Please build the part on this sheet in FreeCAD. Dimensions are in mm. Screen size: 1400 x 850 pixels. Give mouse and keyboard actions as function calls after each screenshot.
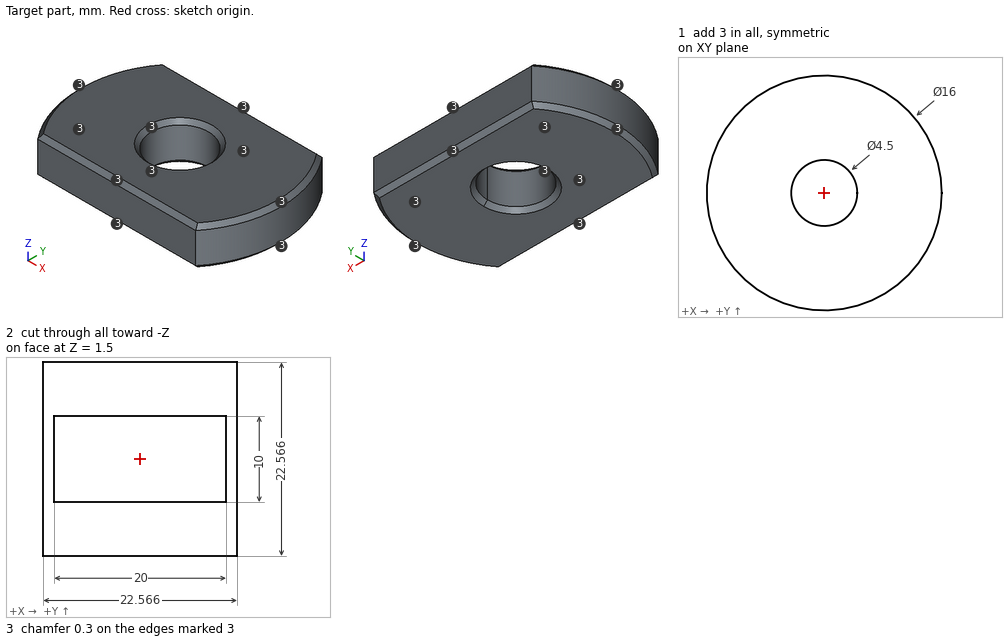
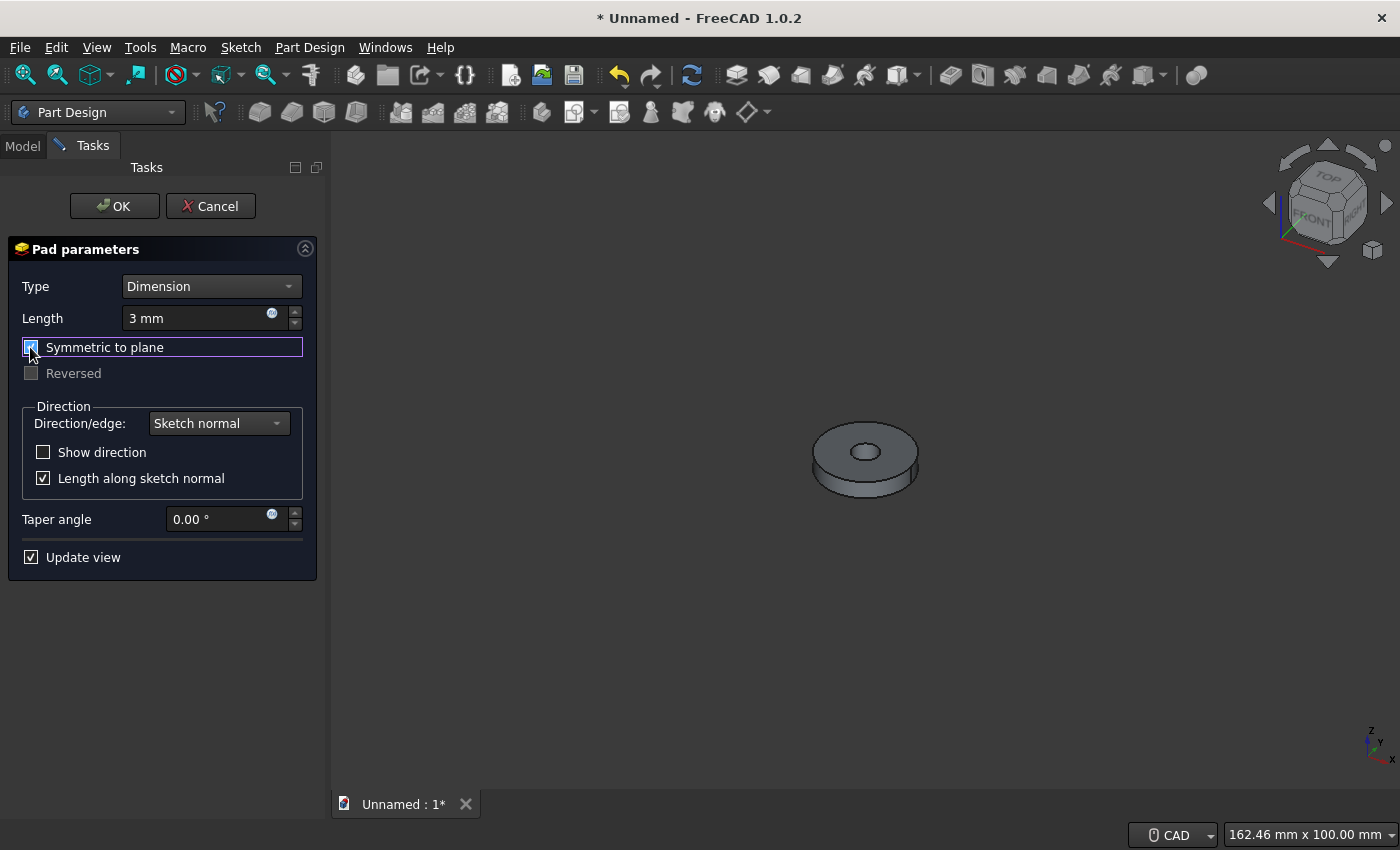
click(115, 206)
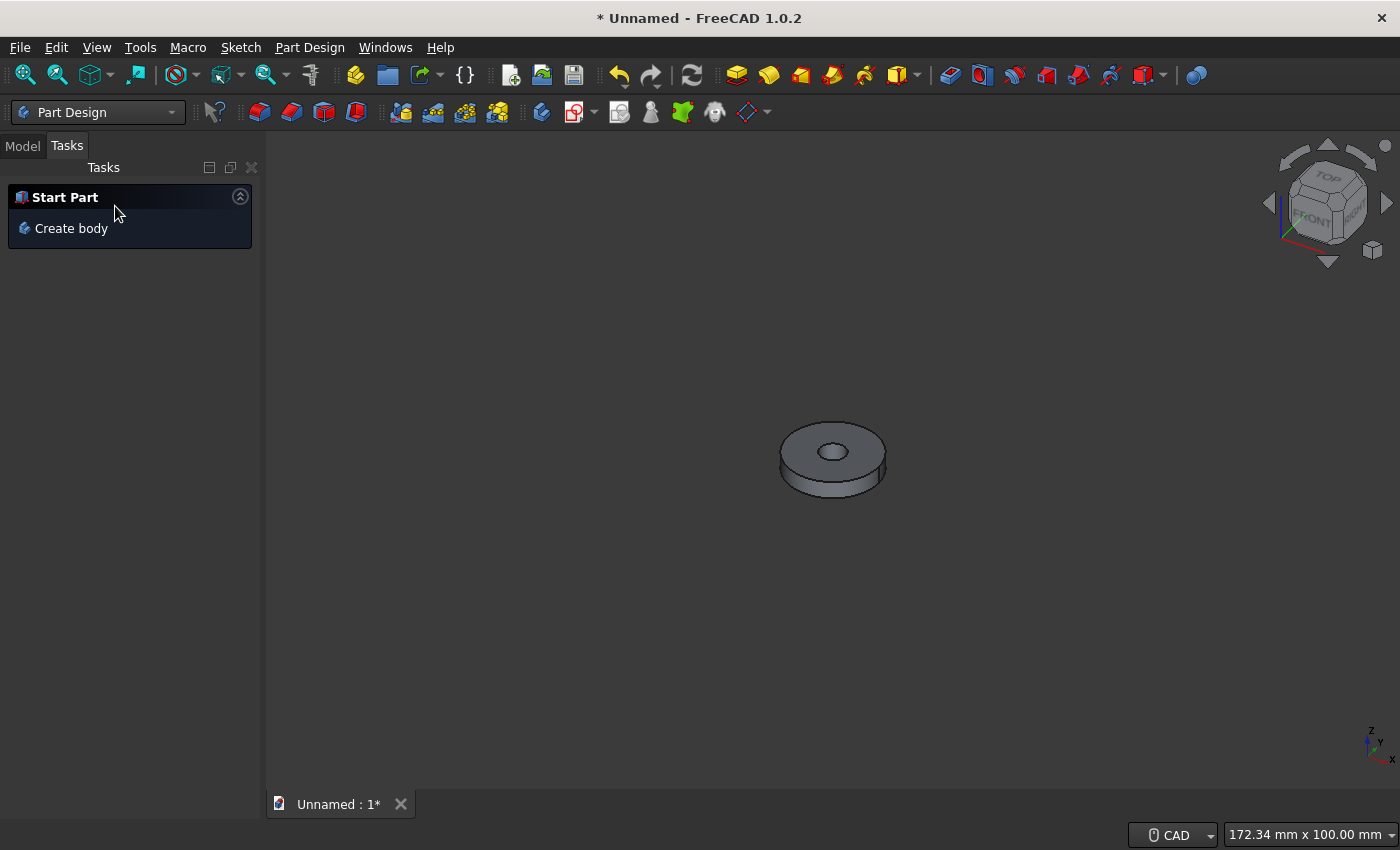
click(26, 76)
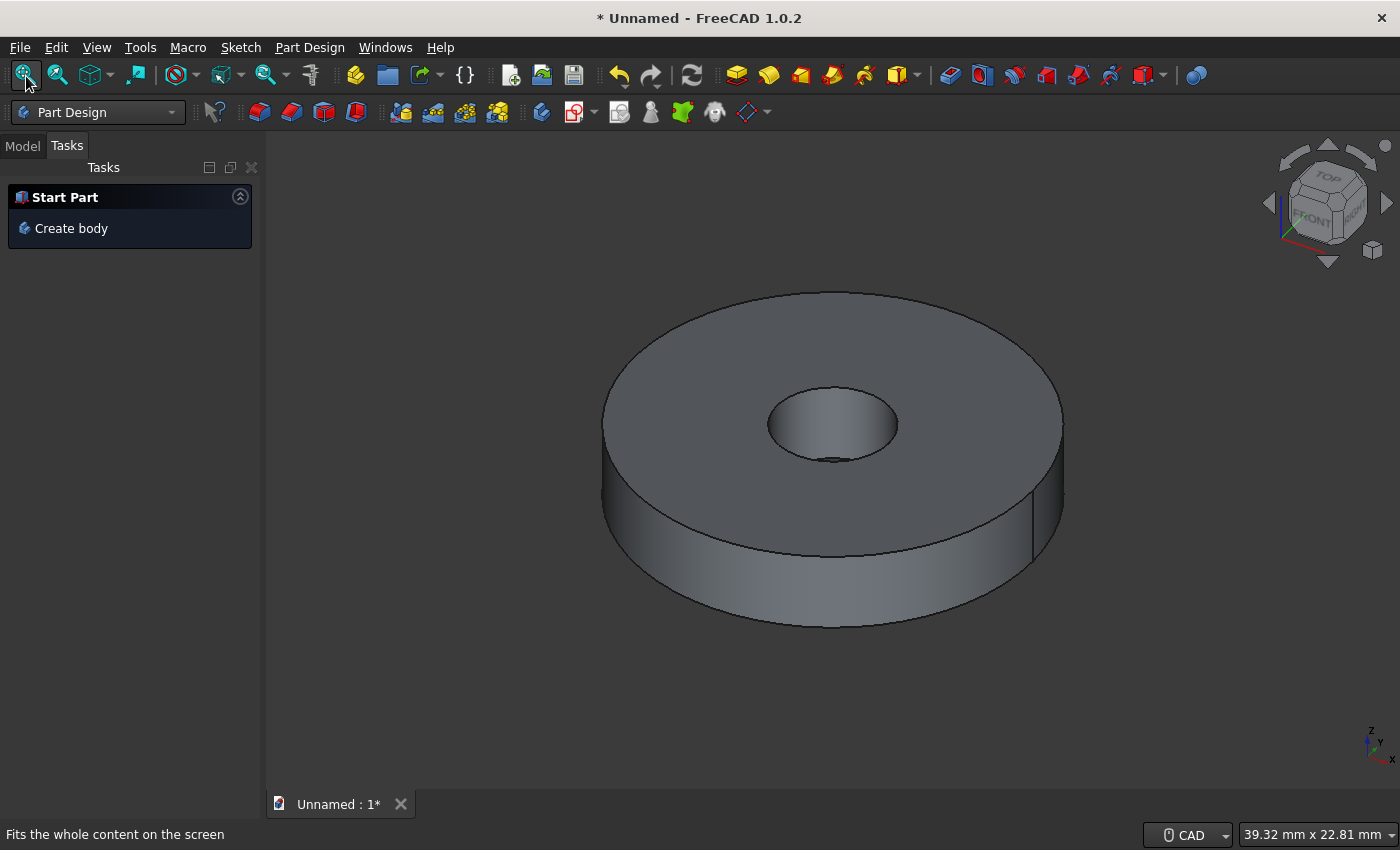
click(956, 377)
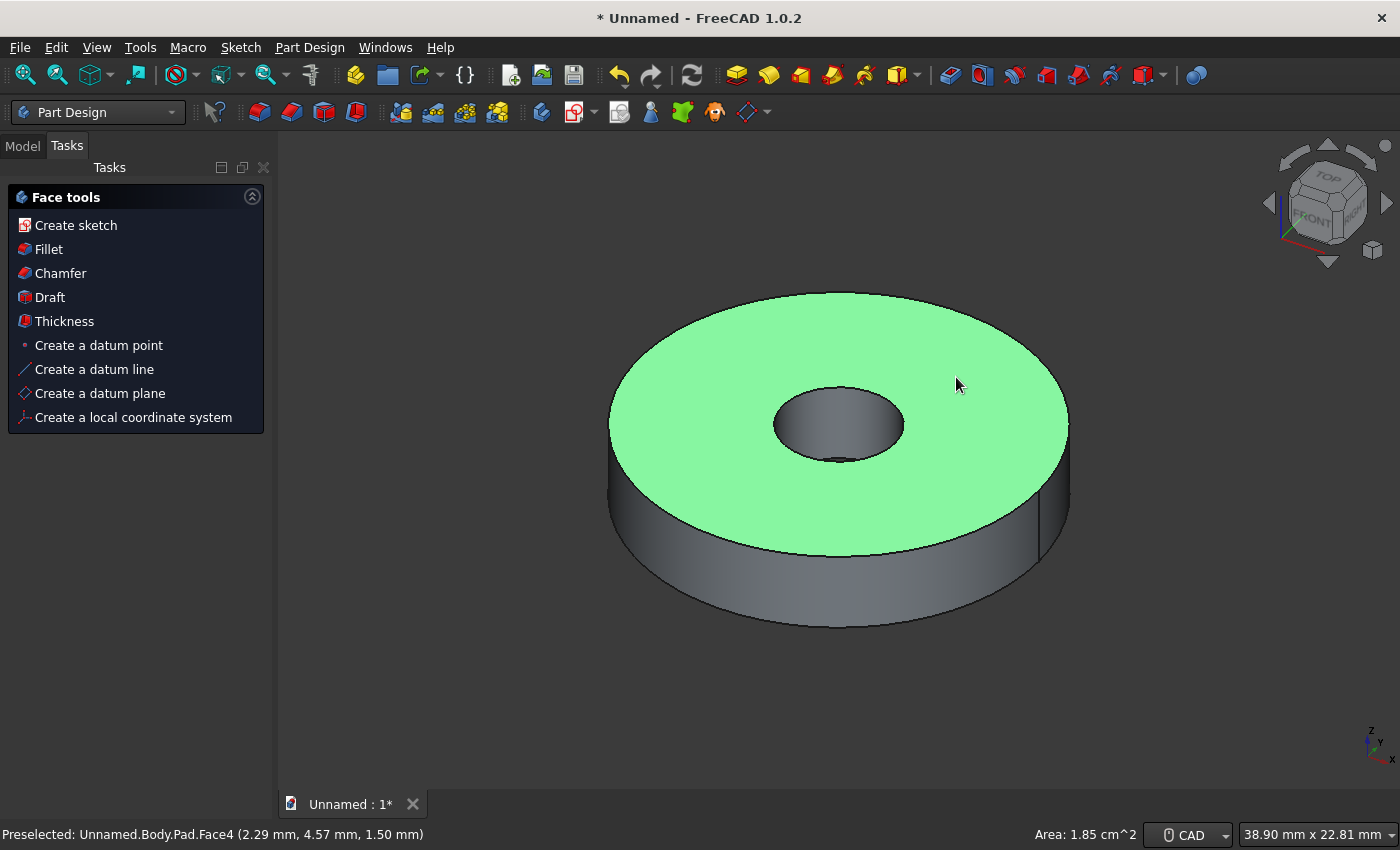
click(574, 112)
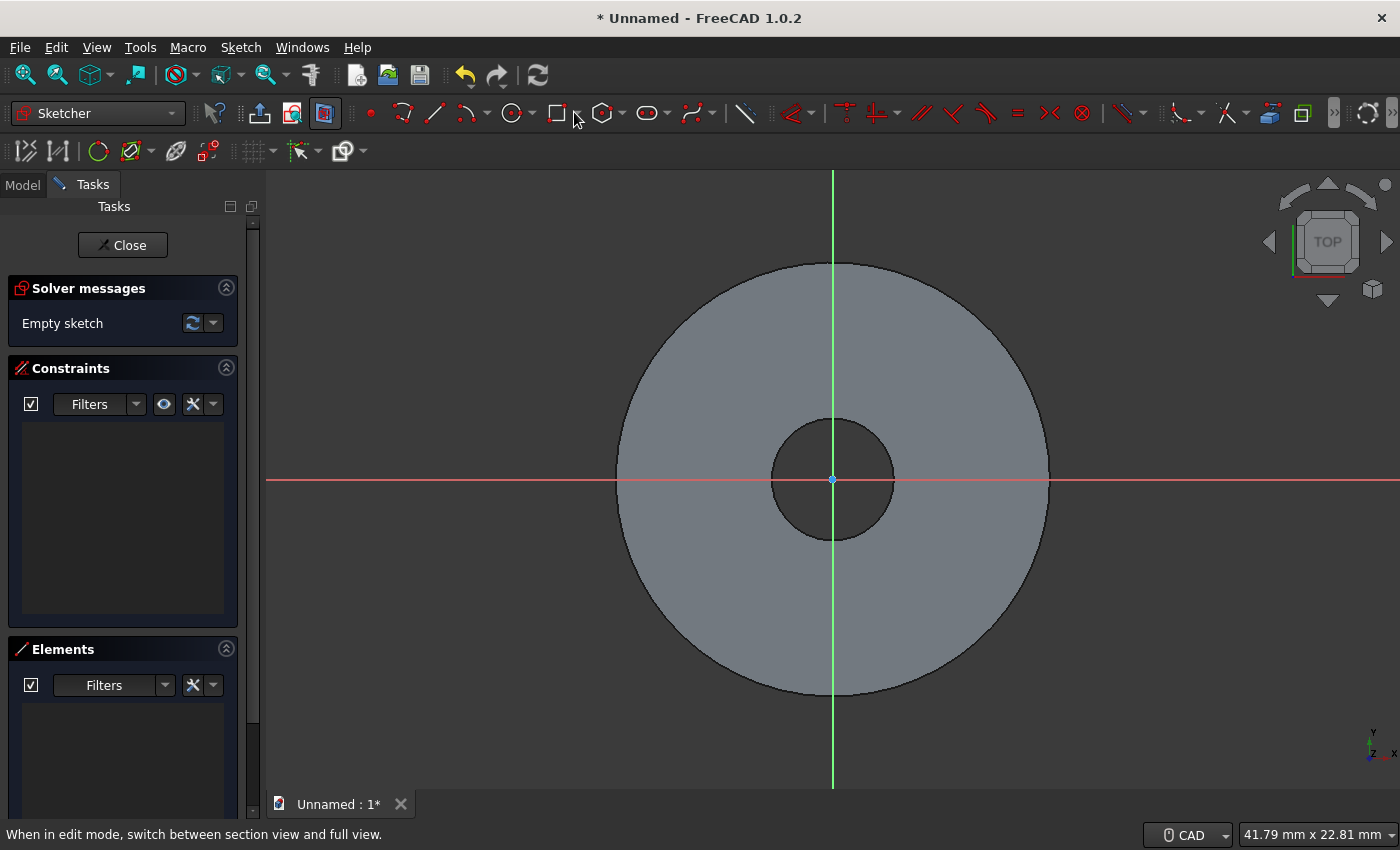
scroll(626, 480, down, 2)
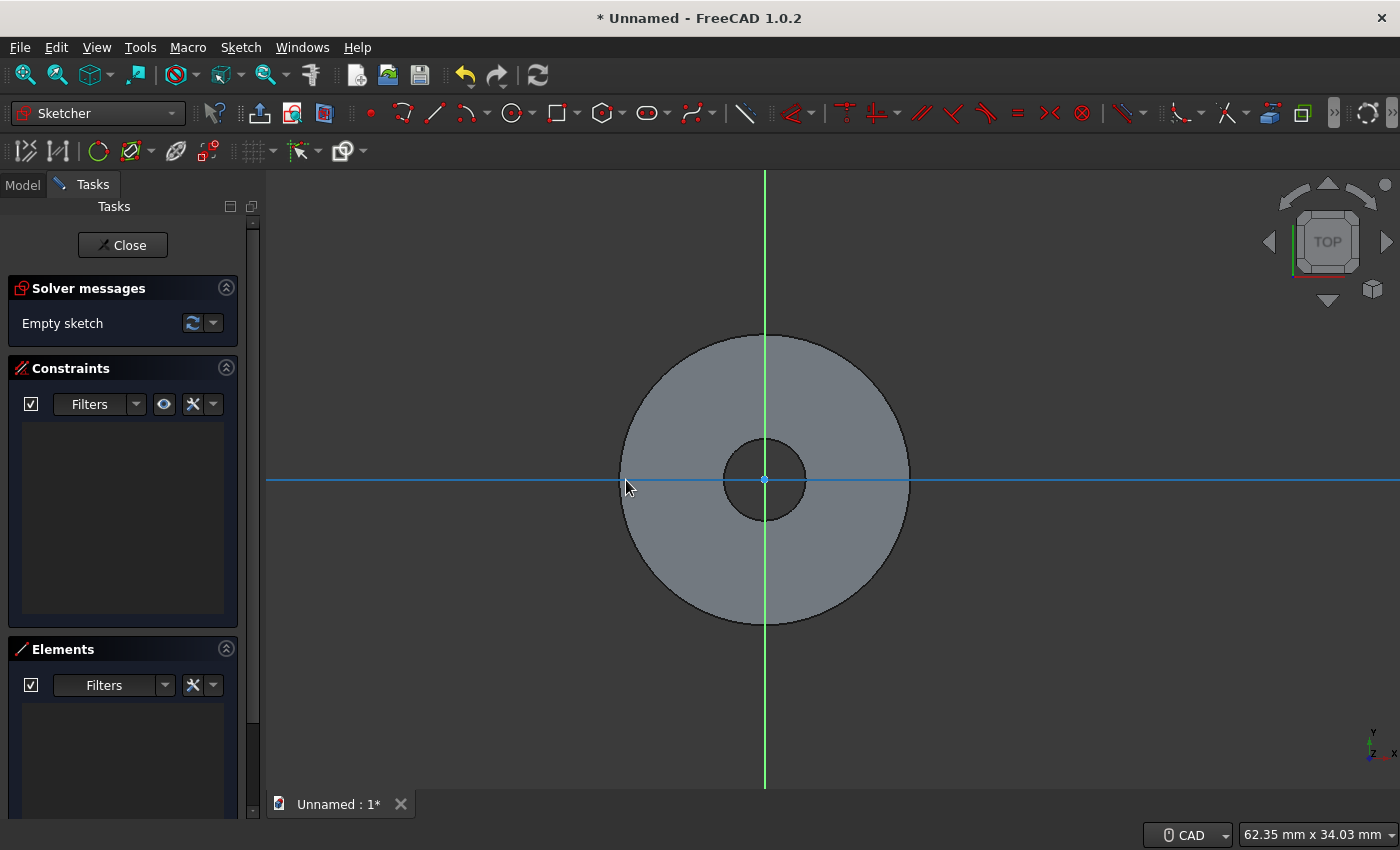
click(580, 114)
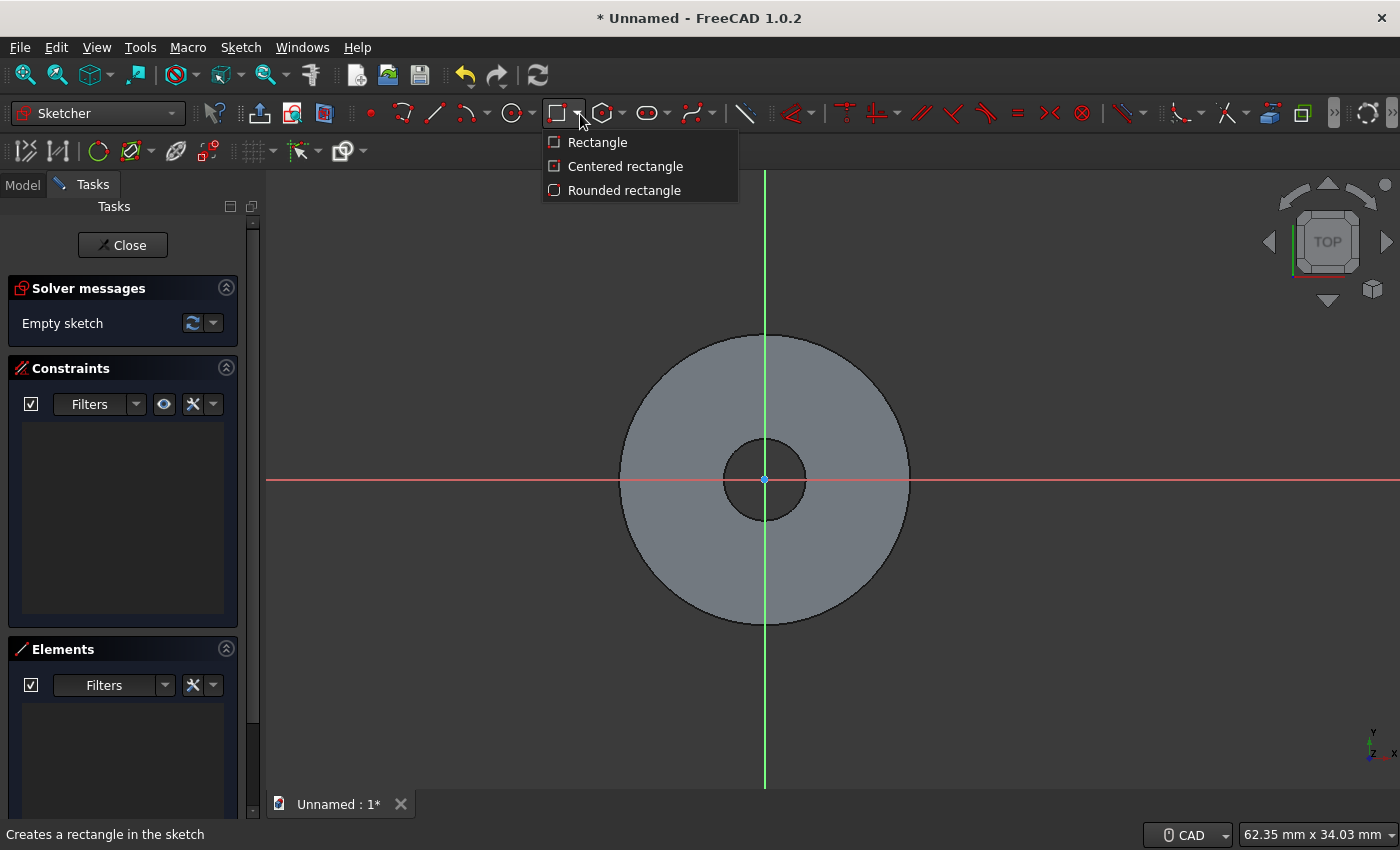
click(640, 166)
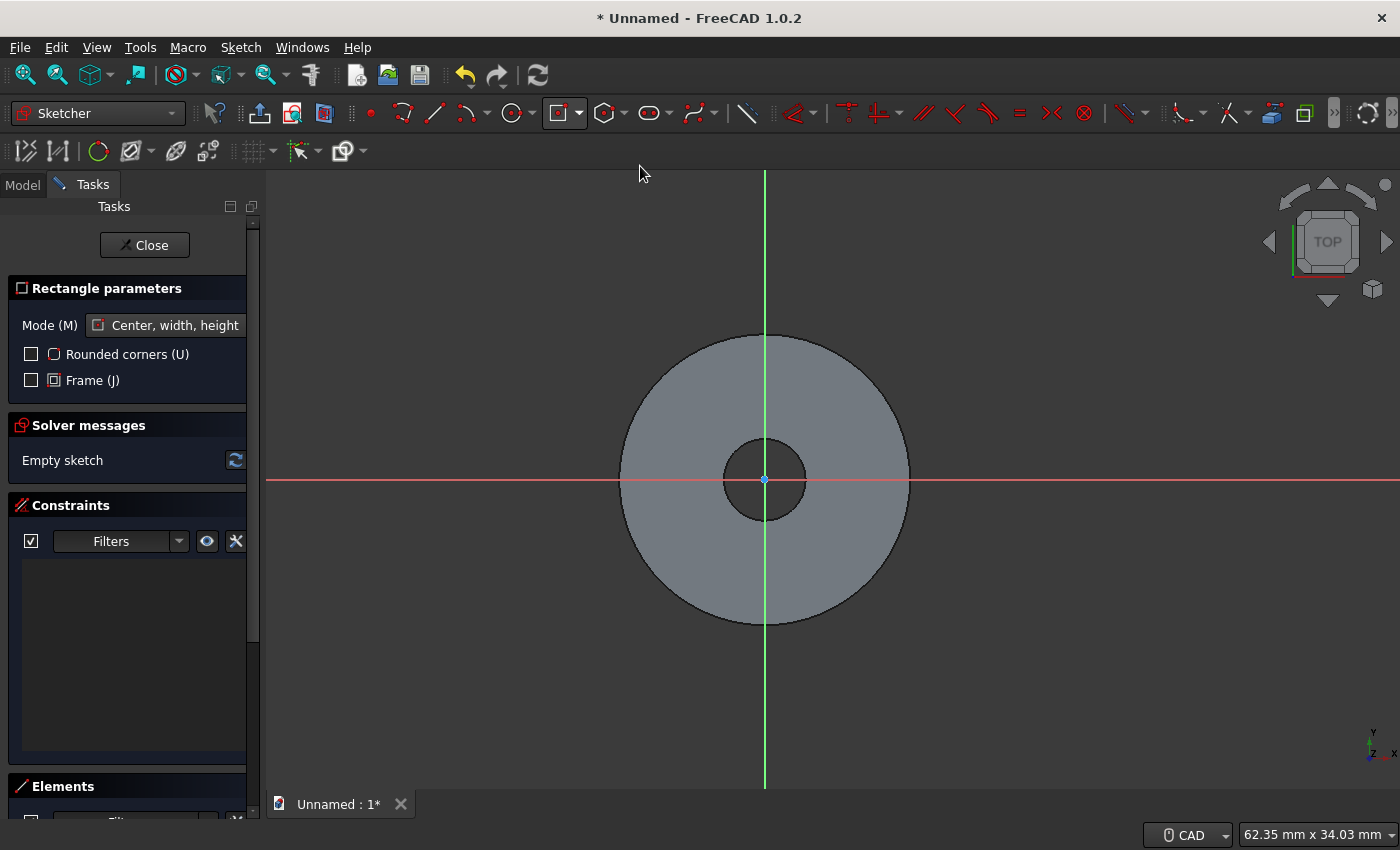
click(765, 480)
click(970, 275)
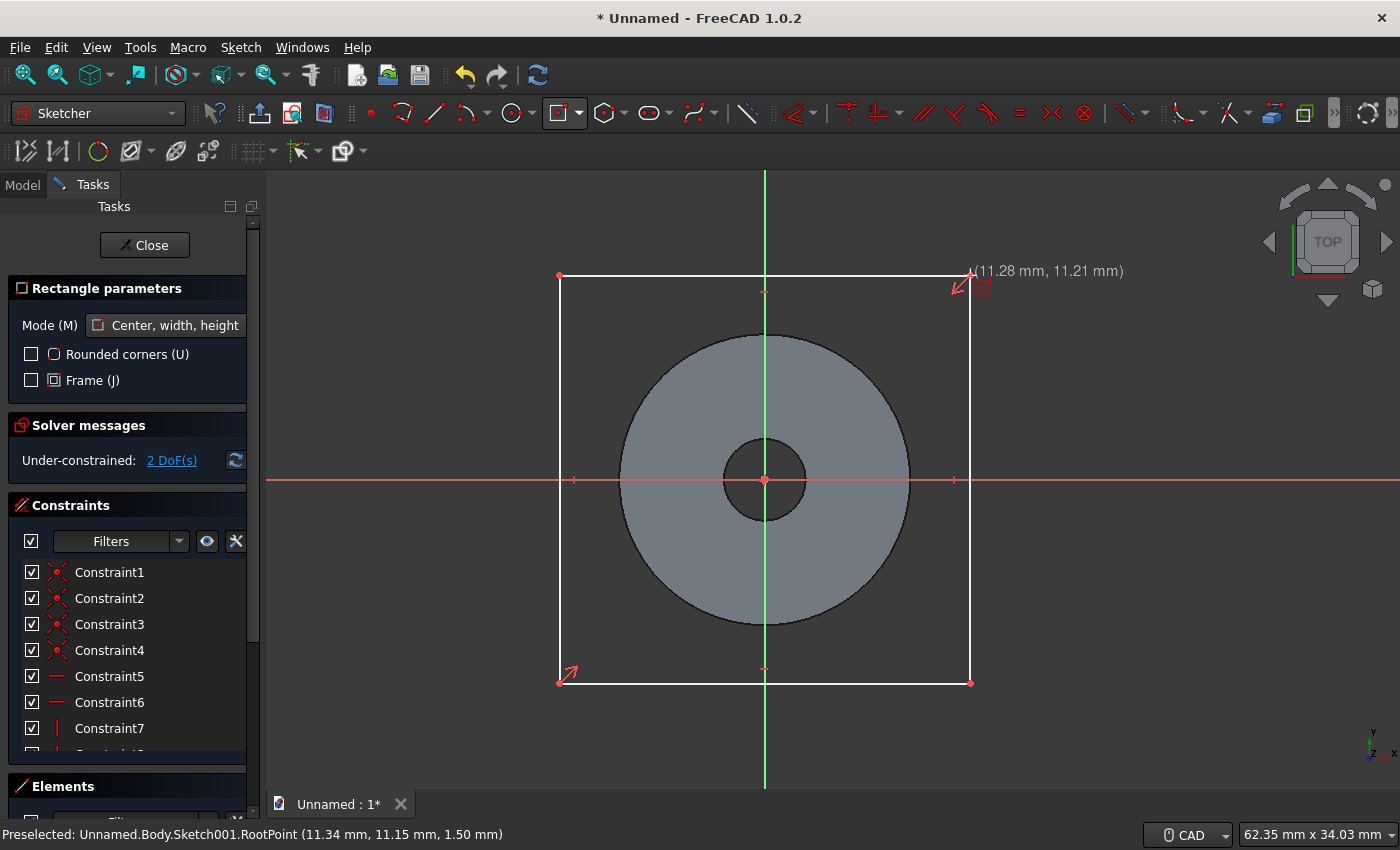
click(765, 480)
click(947, 389)
key(Escape)